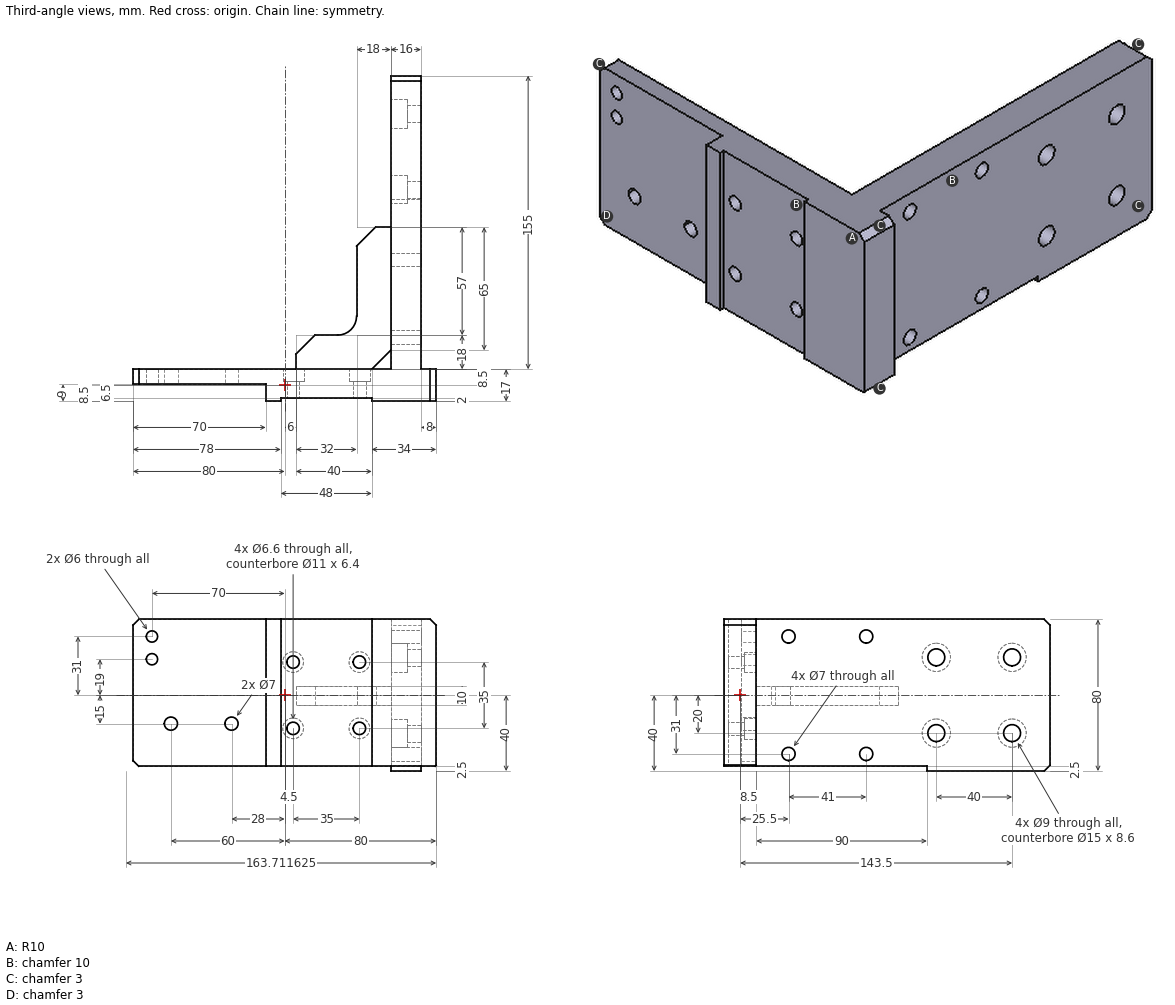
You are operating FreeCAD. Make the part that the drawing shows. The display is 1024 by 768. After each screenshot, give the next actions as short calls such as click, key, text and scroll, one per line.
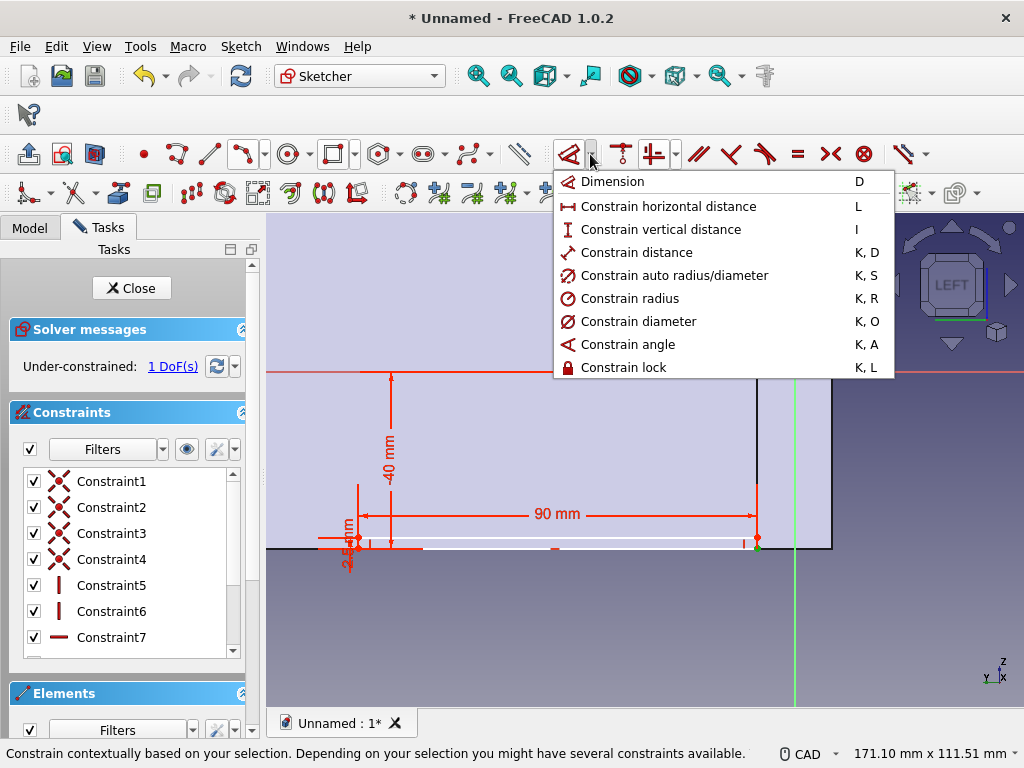
click(724, 206)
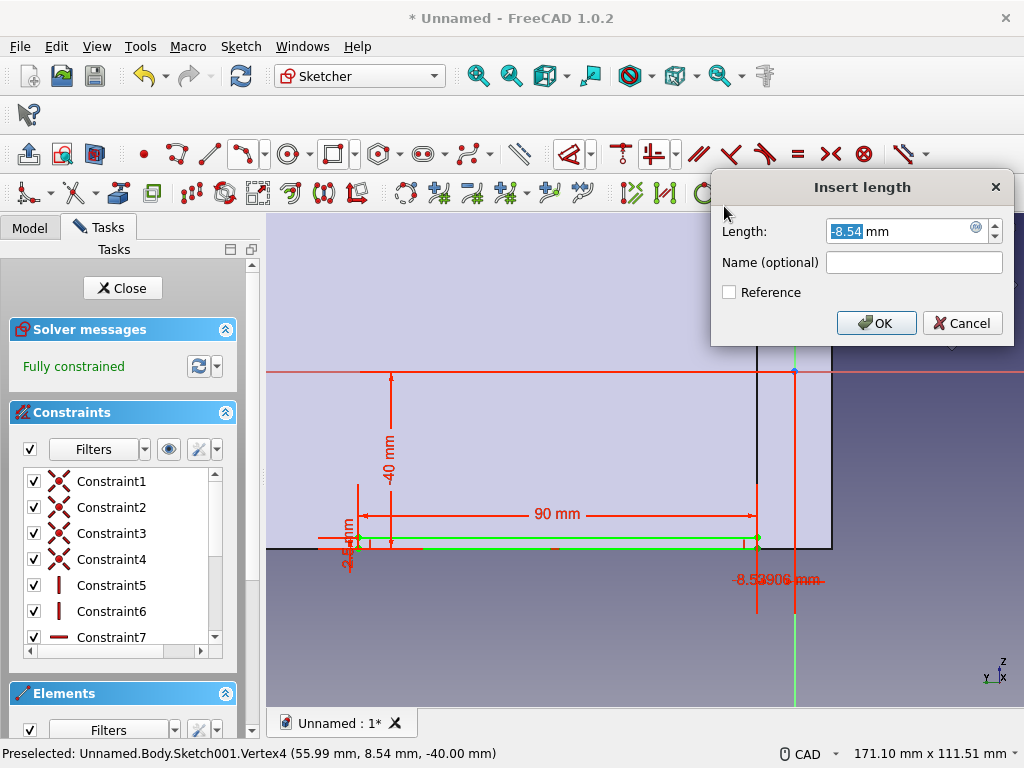
text(-8.5)
key(Return)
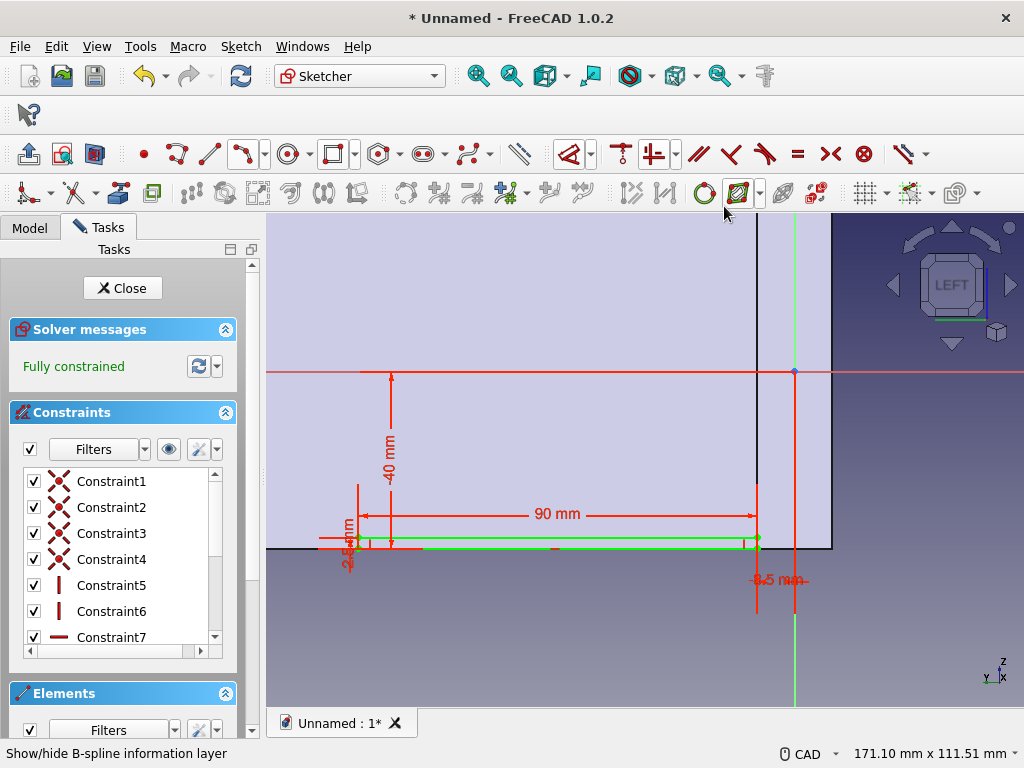
click(123, 288)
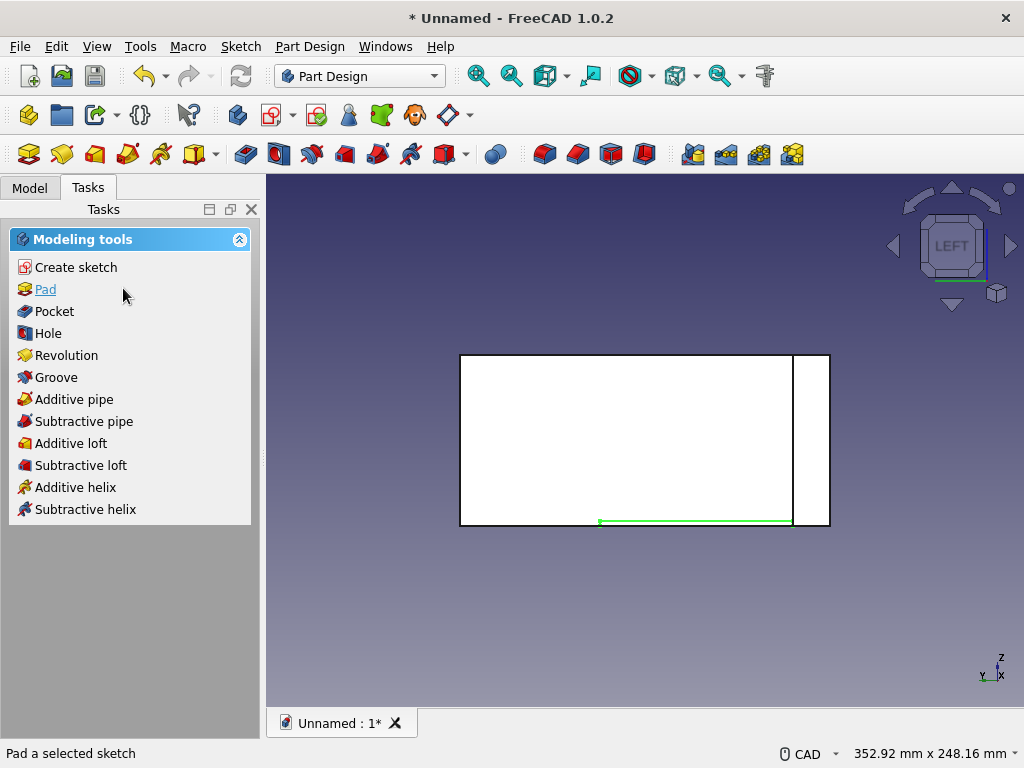
click(246, 154)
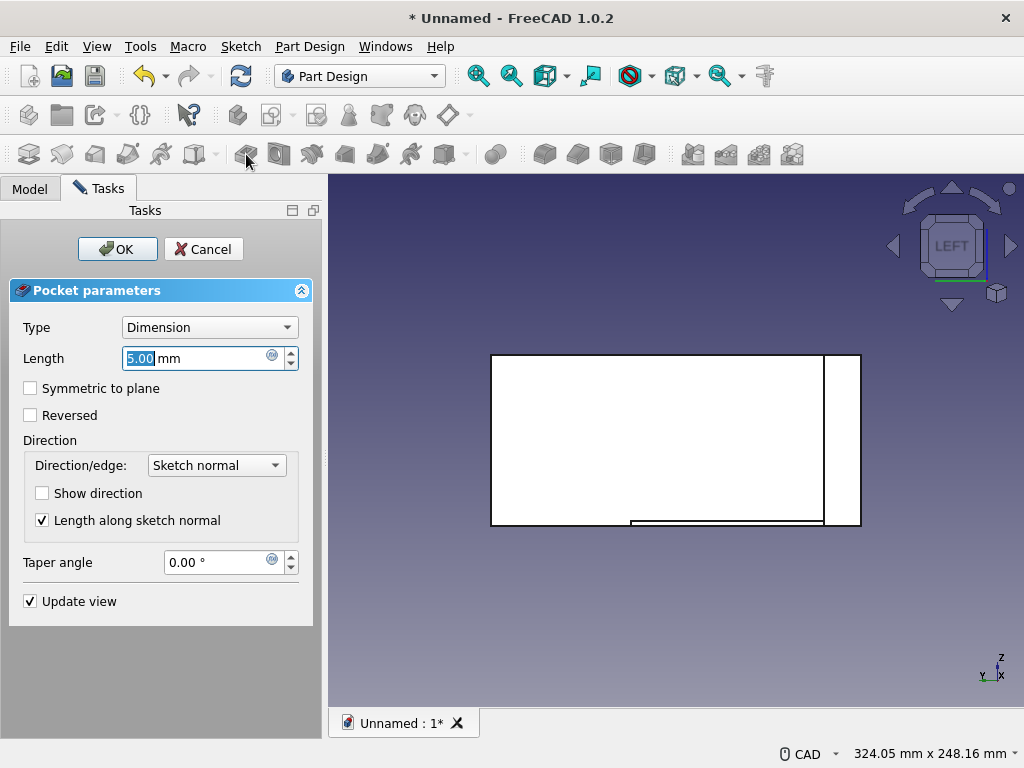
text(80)
key(Tab)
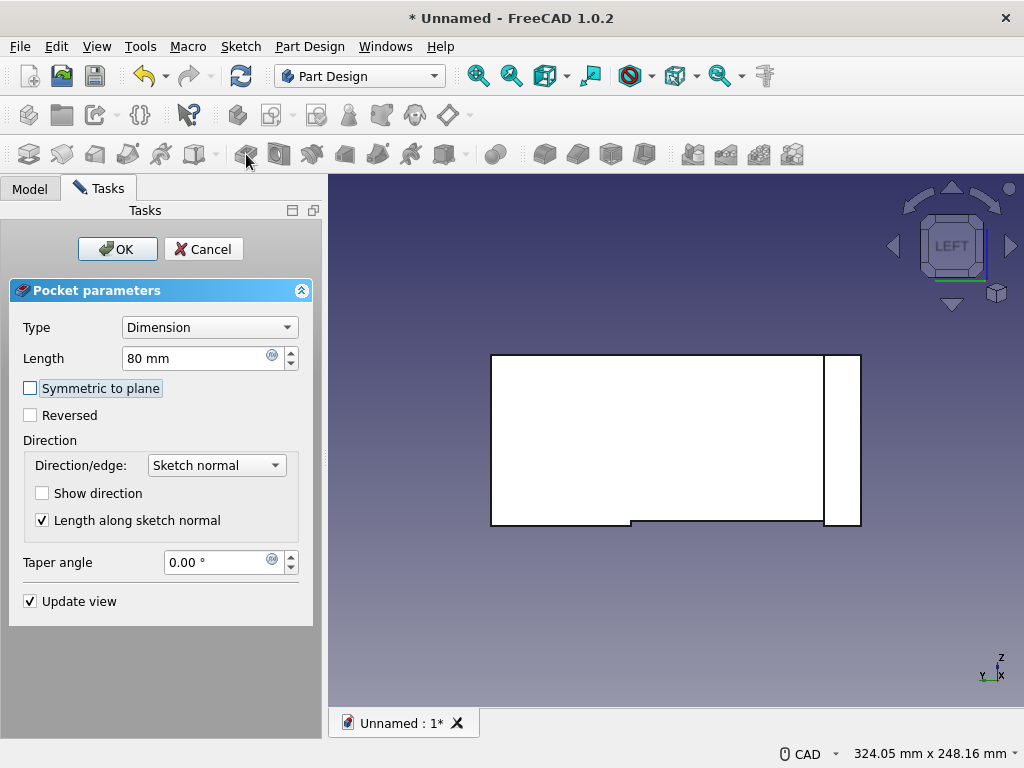
click(118, 249)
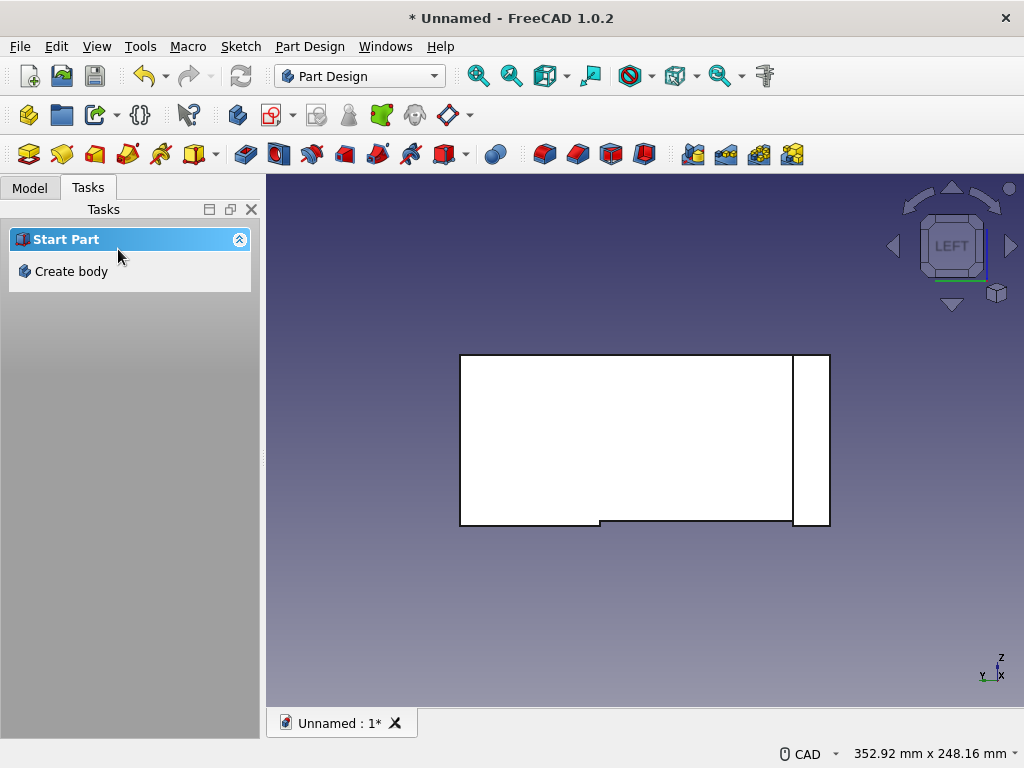
click(270, 116)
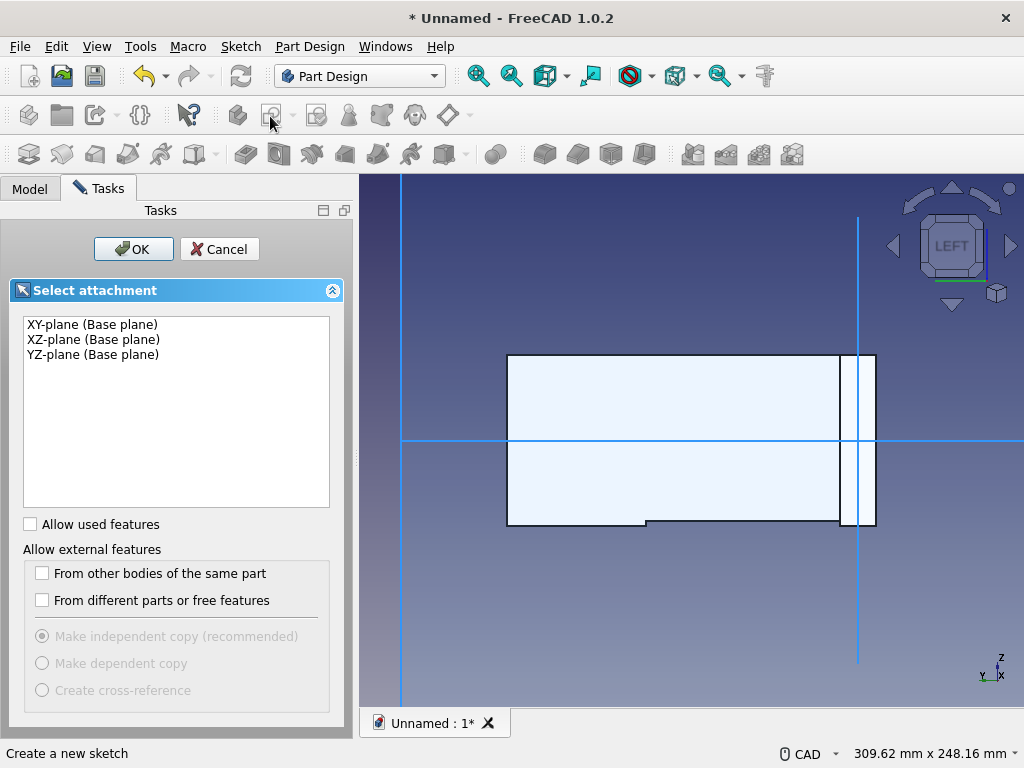
click(84, 324)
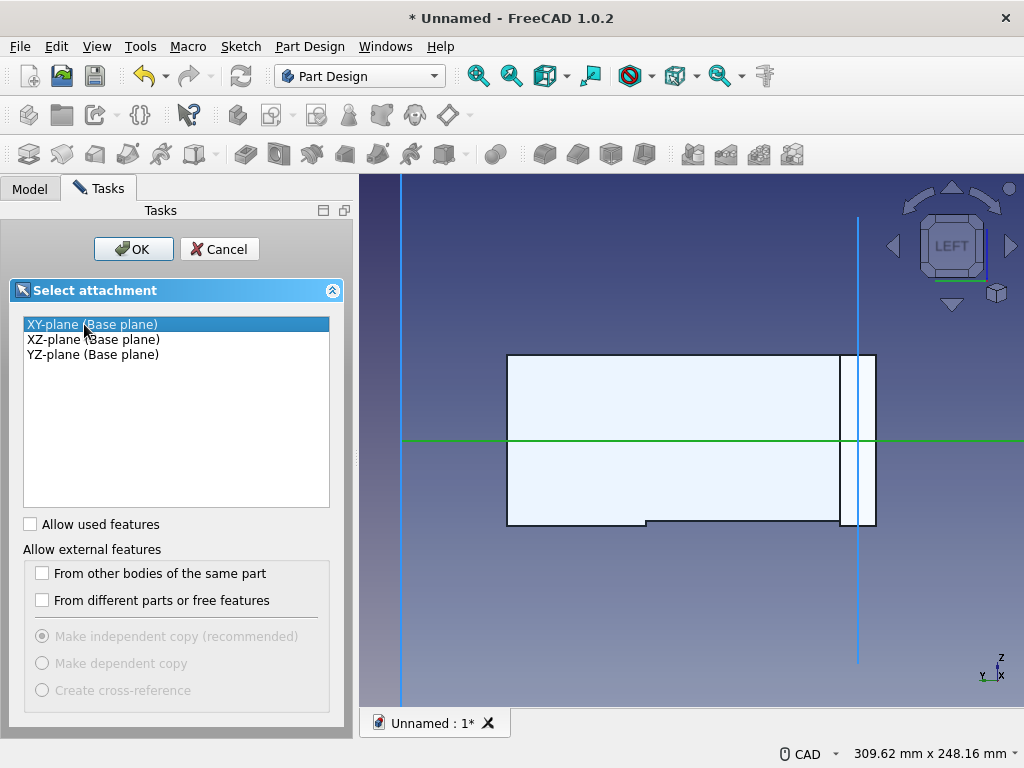
click(134, 249)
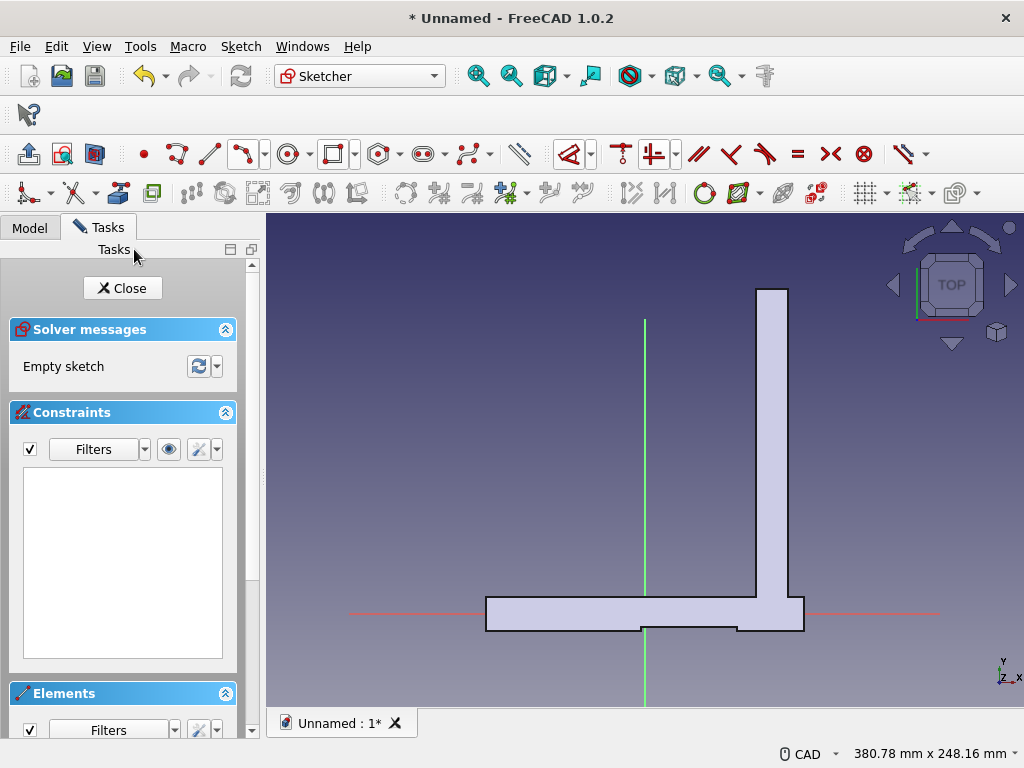
click(95, 154)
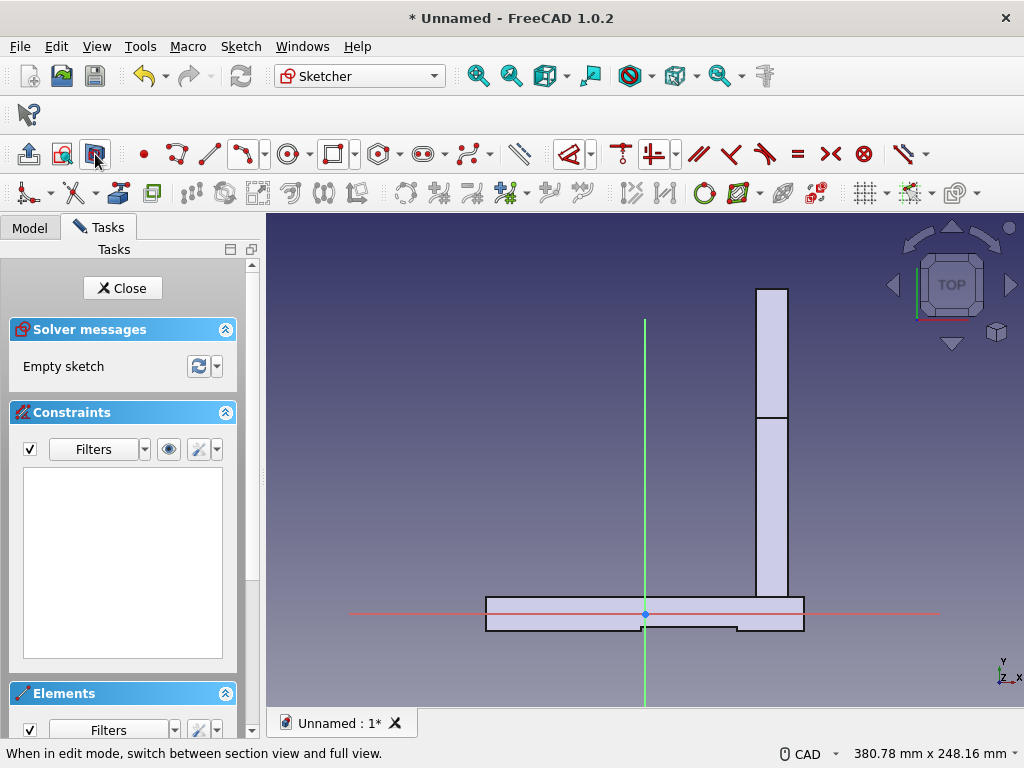
scroll(852, 618, up, 3)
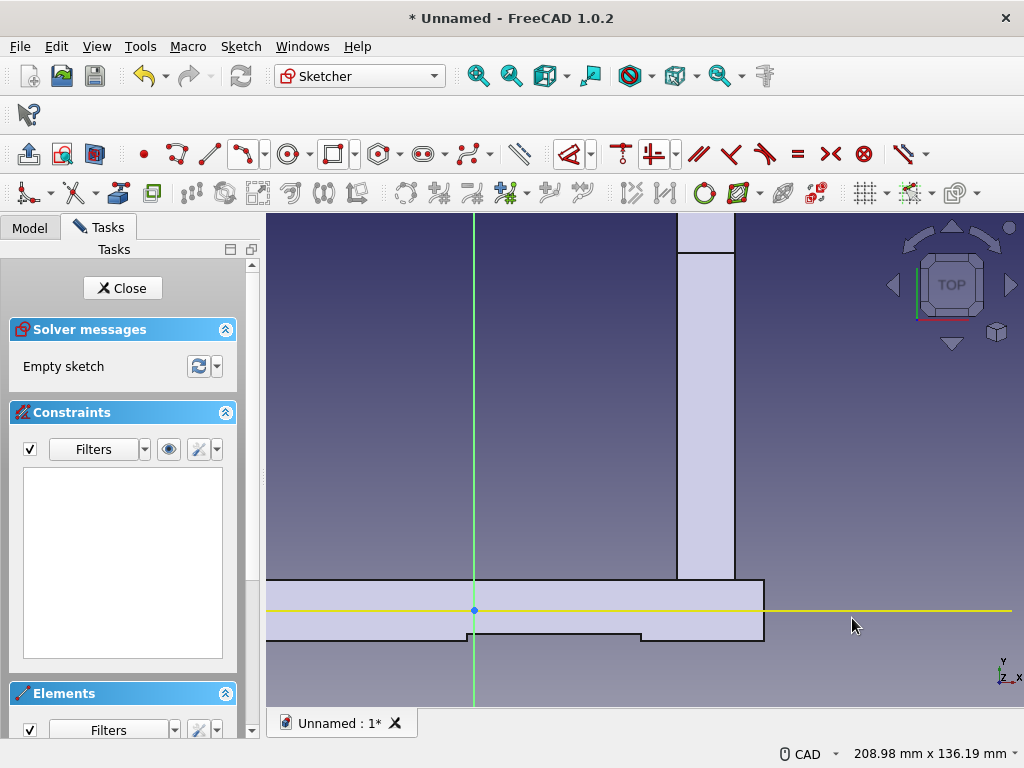
key(g)
key(m)